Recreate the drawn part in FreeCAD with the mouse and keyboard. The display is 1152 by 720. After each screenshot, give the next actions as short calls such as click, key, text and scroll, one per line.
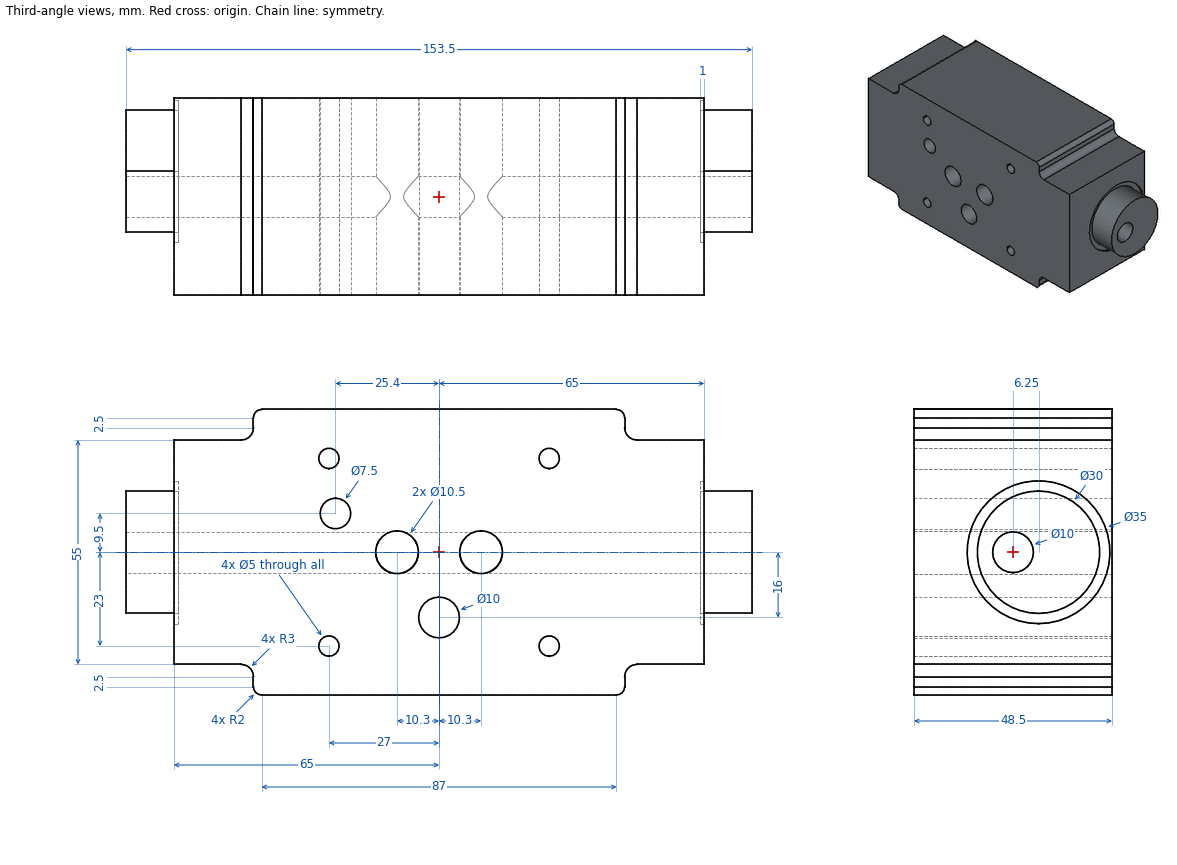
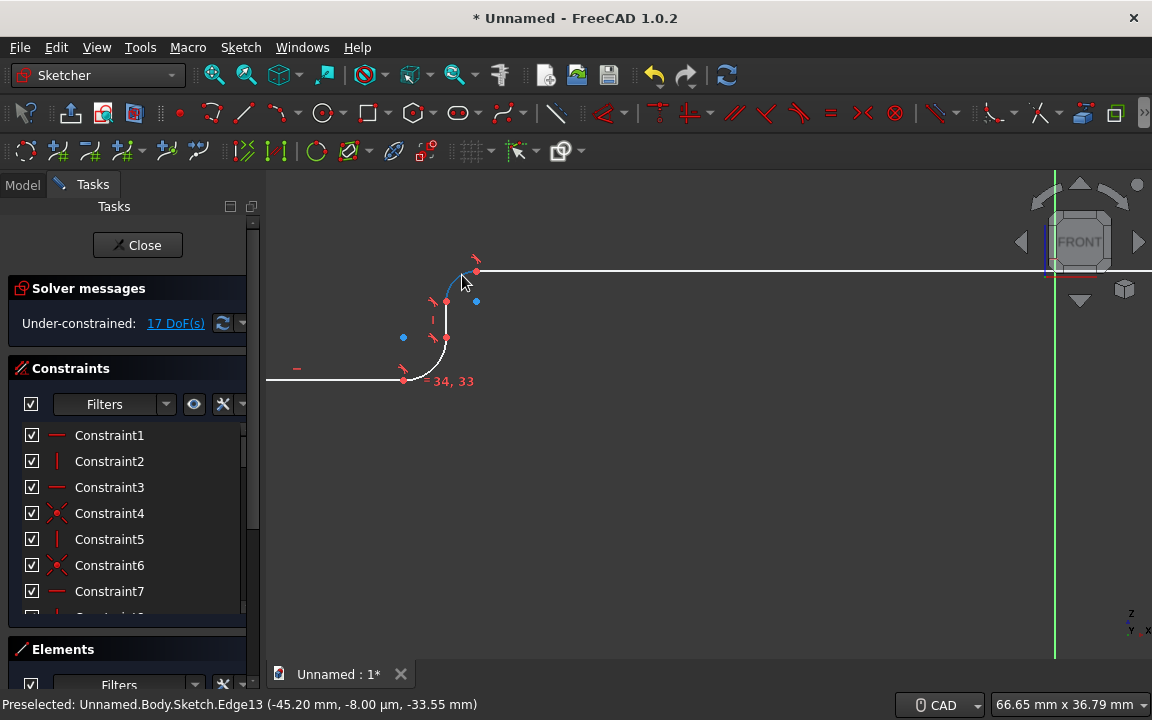
click(463, 274)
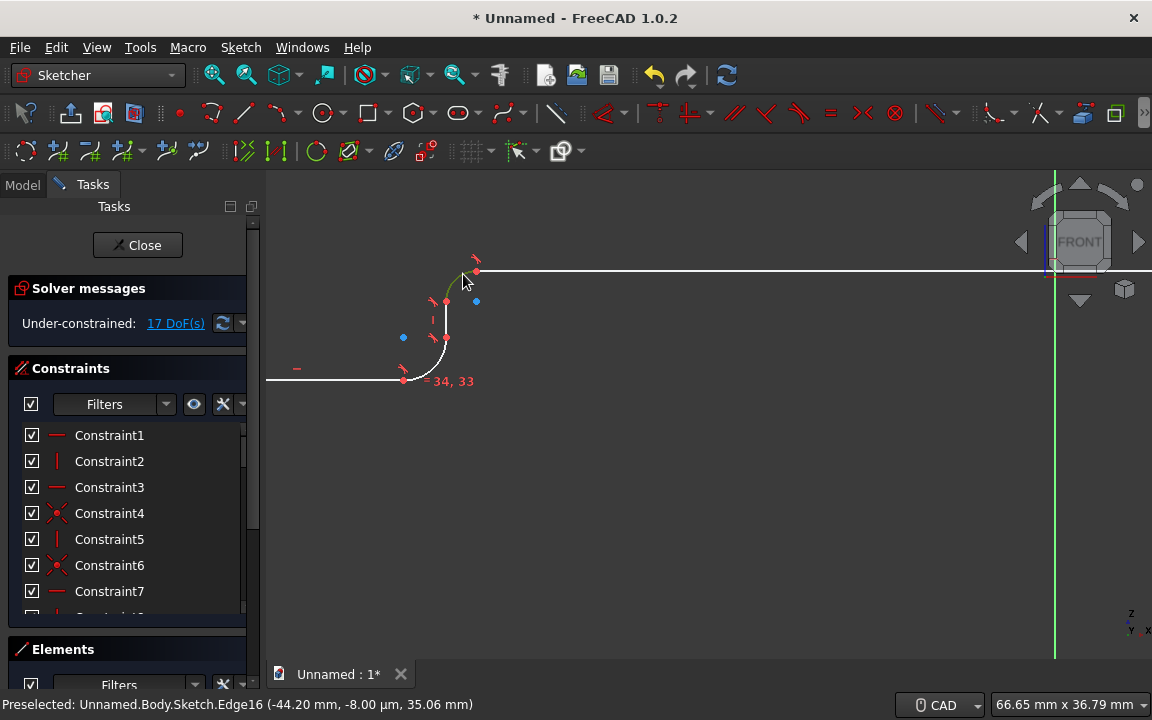
scroll(462, 275, down, 6)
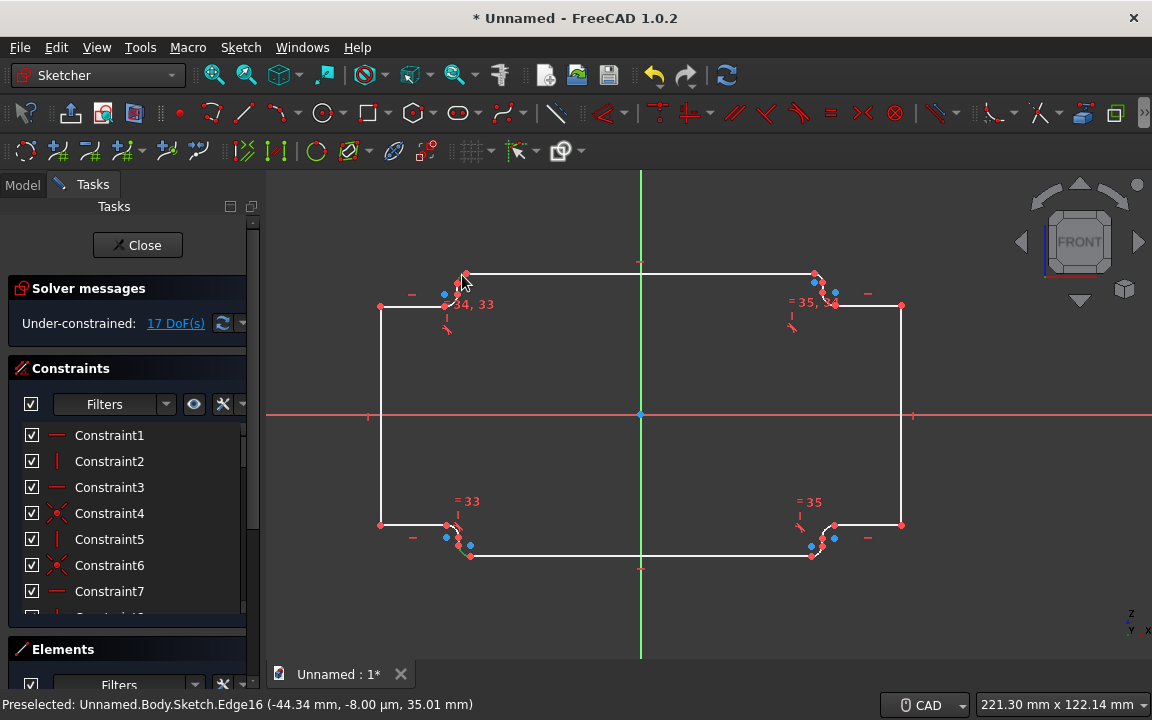
scroll(822, 278, up, 7)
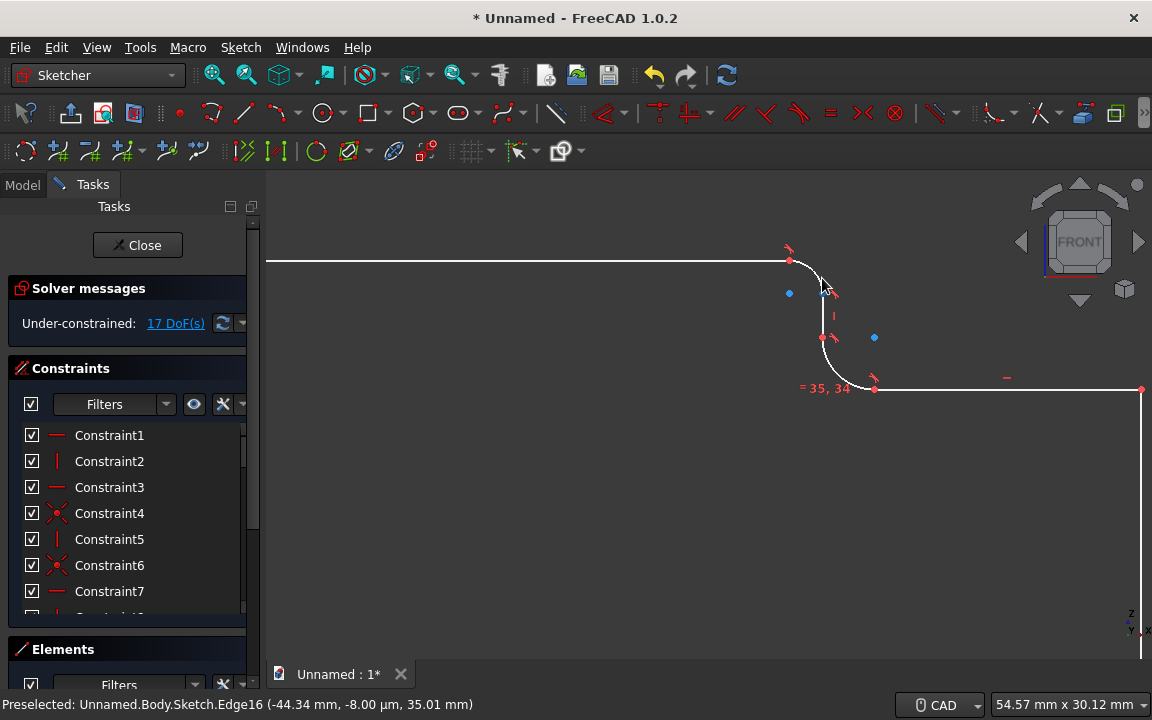
click(819, 279)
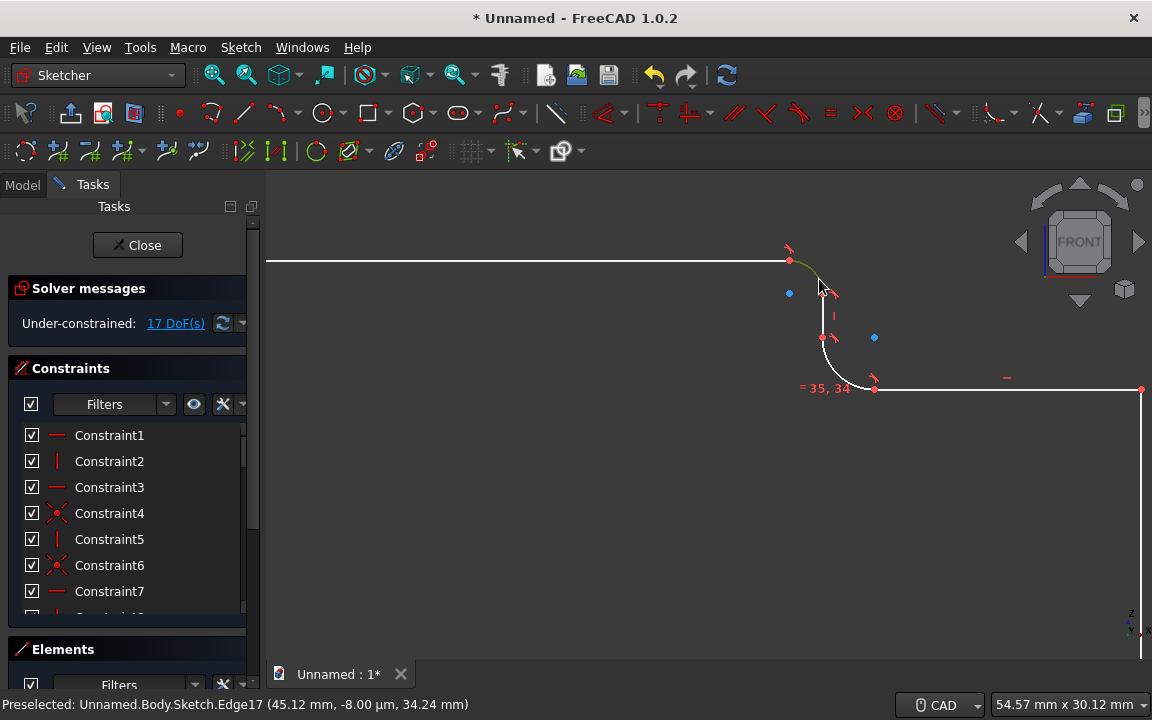
scroll(822, 278, down, 7)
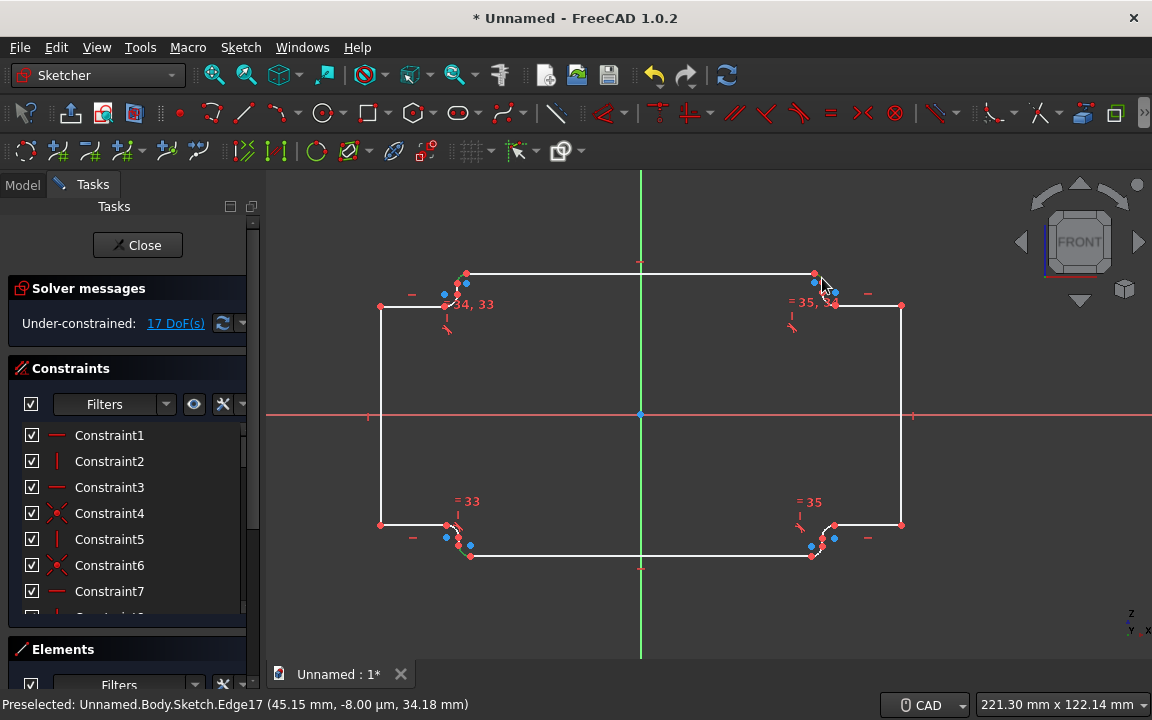
scroll(817, 555, up, 6)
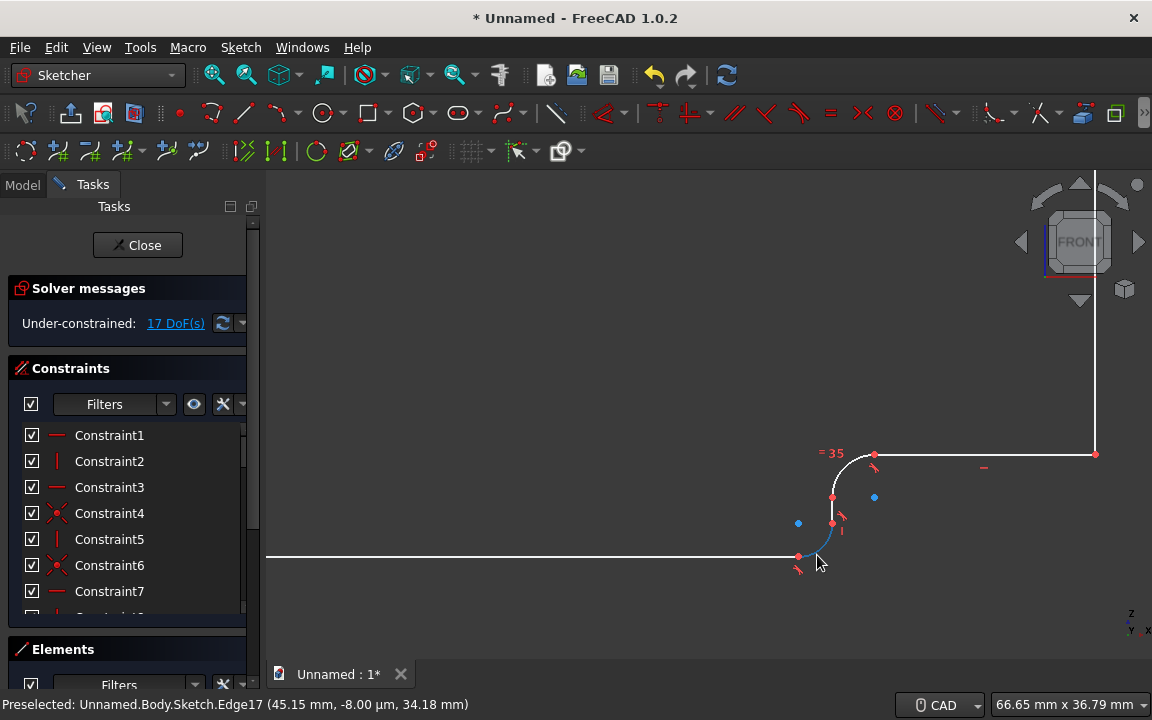
click(814, 553)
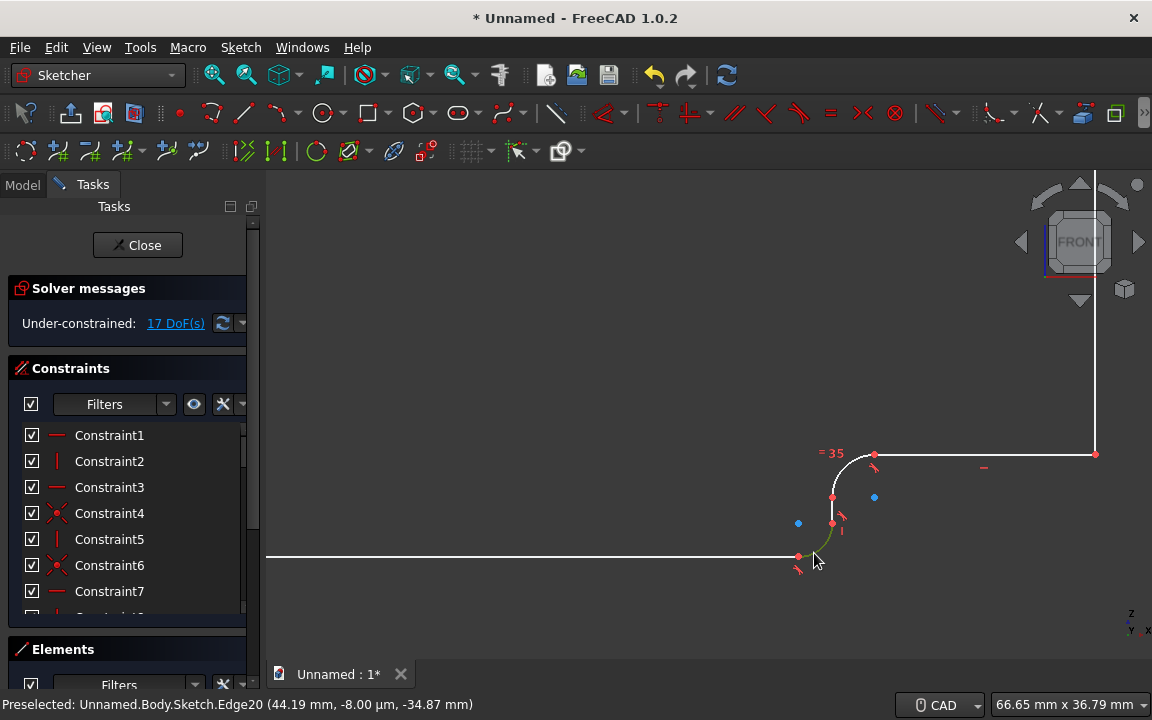
click(832, 114)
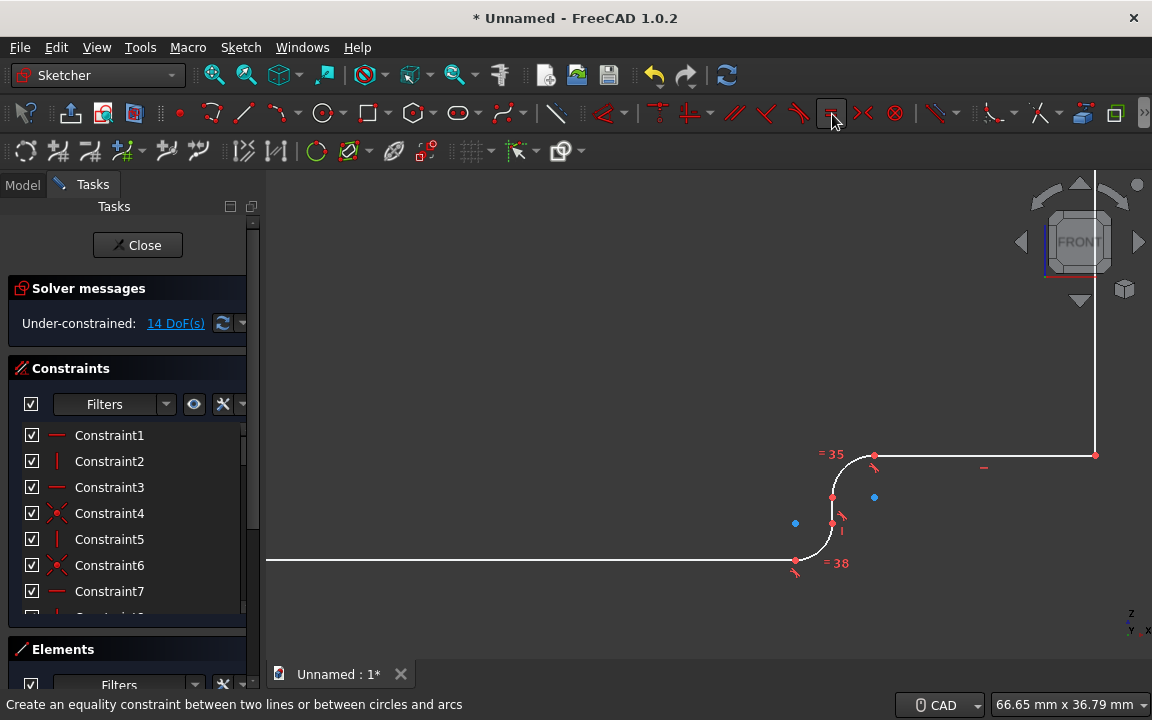
scroll(817, 555, down, 6)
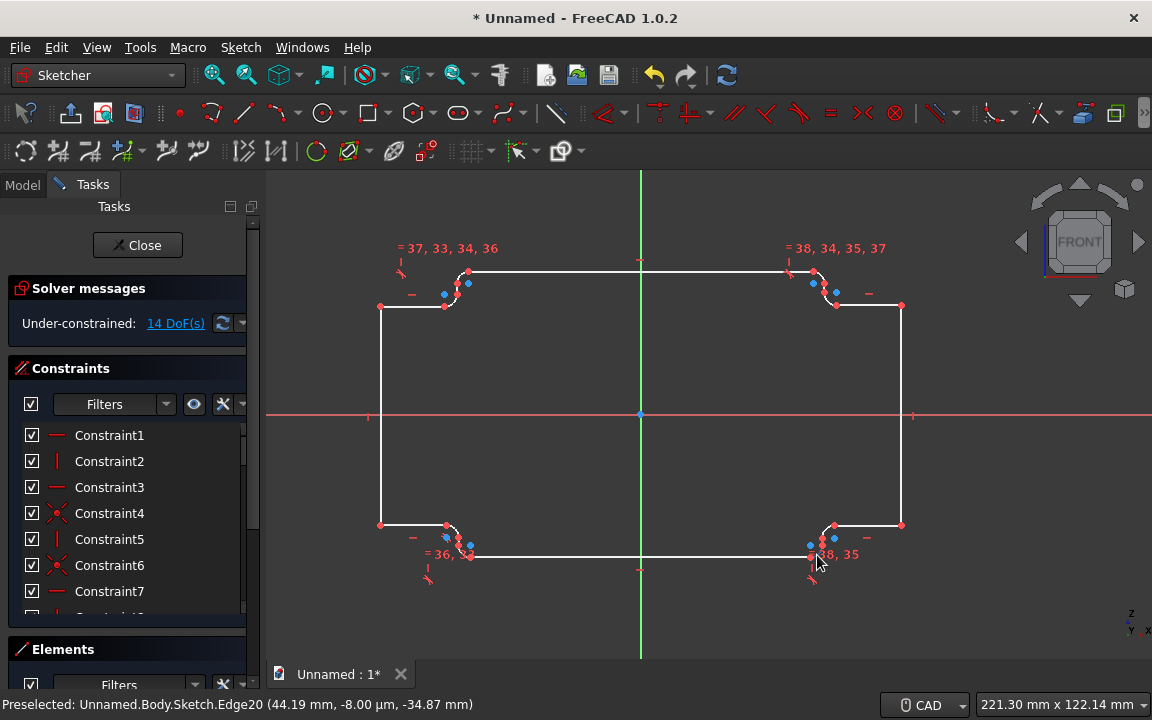
click(446, 538)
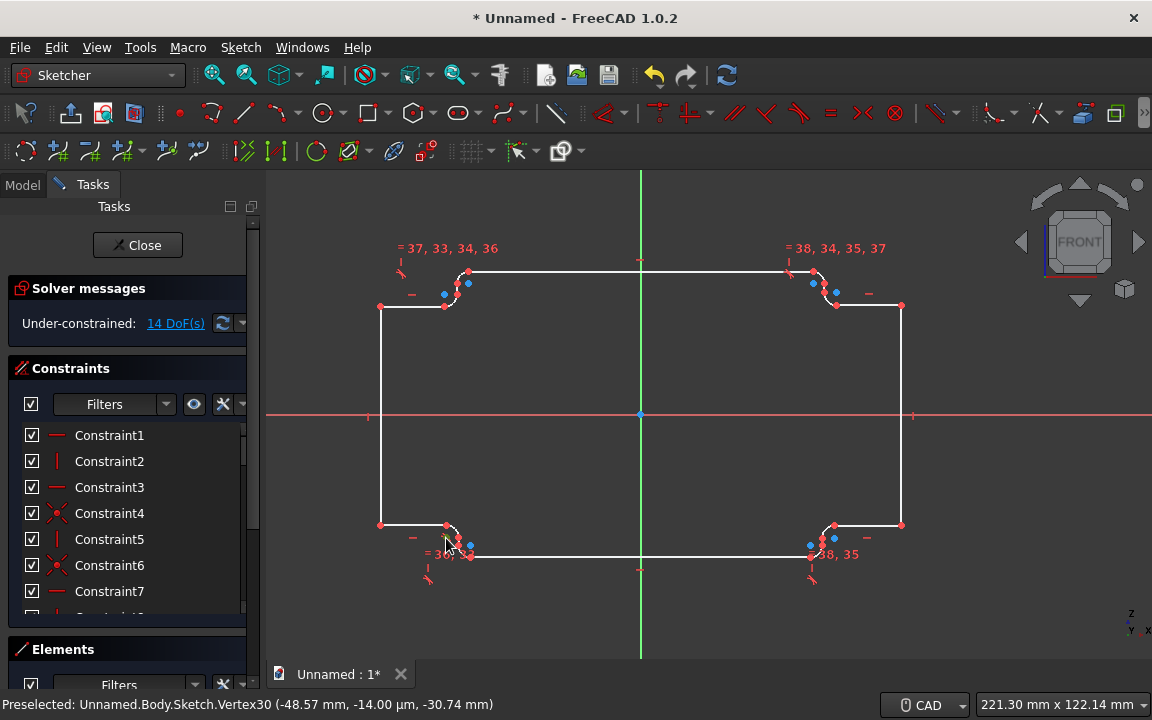
click(445, 294)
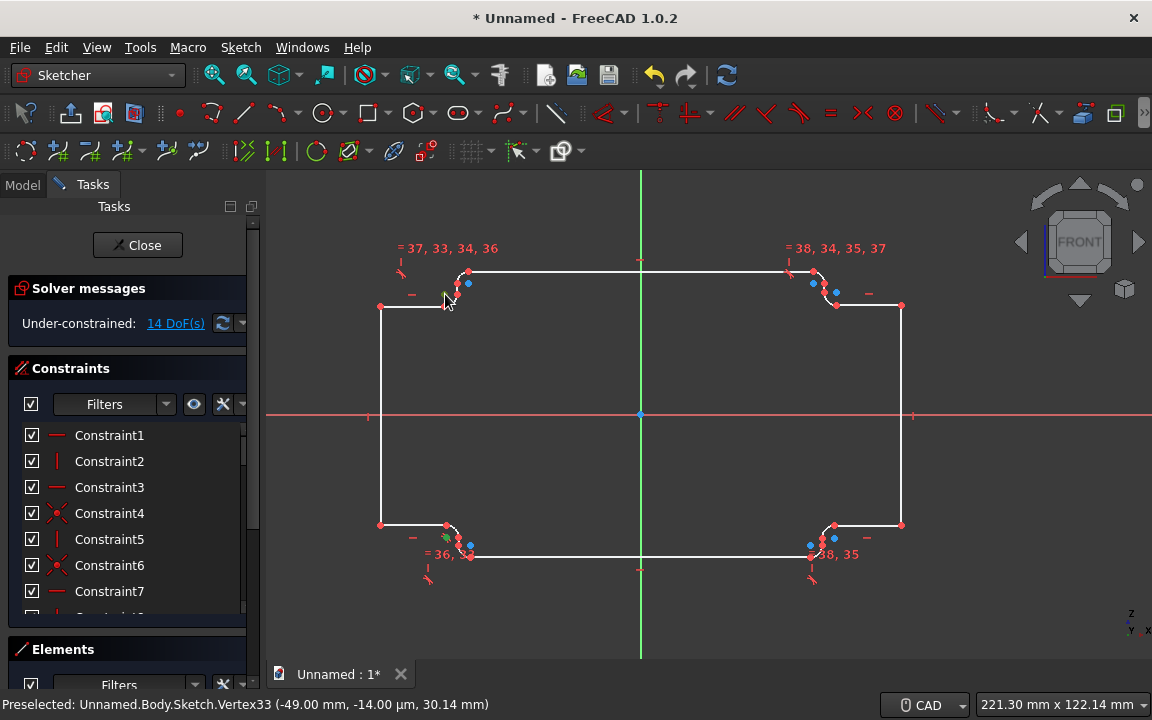
click(344, 415)